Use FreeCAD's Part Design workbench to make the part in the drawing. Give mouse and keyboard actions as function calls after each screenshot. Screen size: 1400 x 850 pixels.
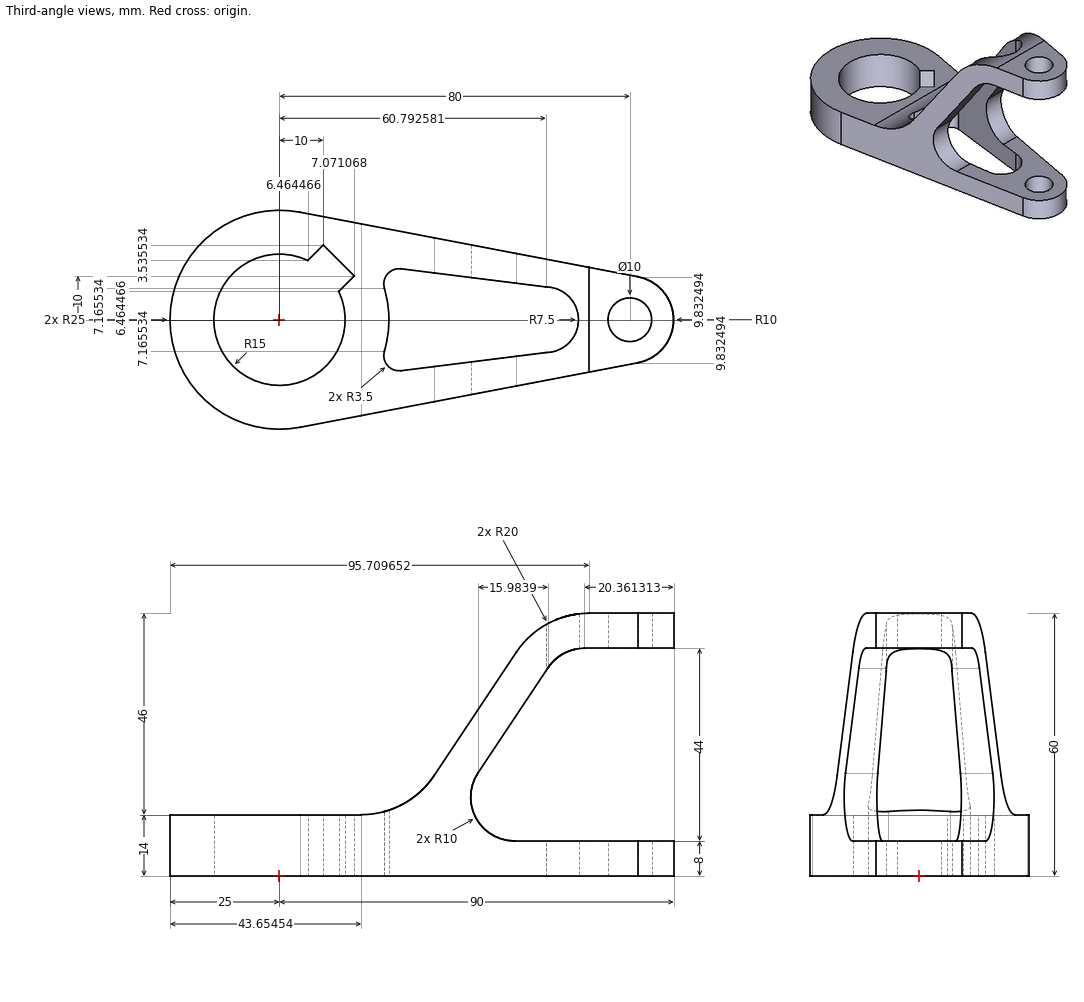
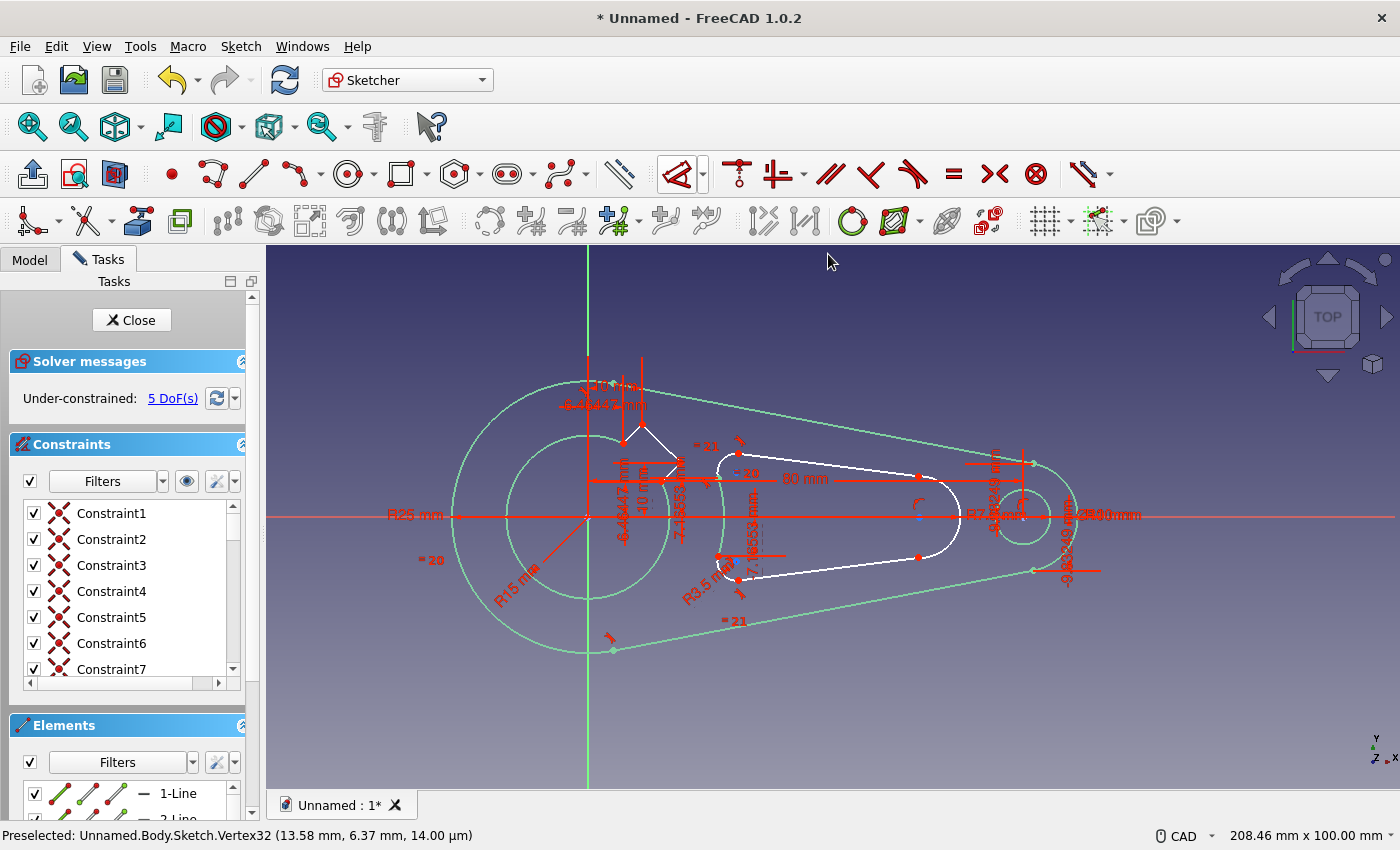
scroll(631, 436, up, 4)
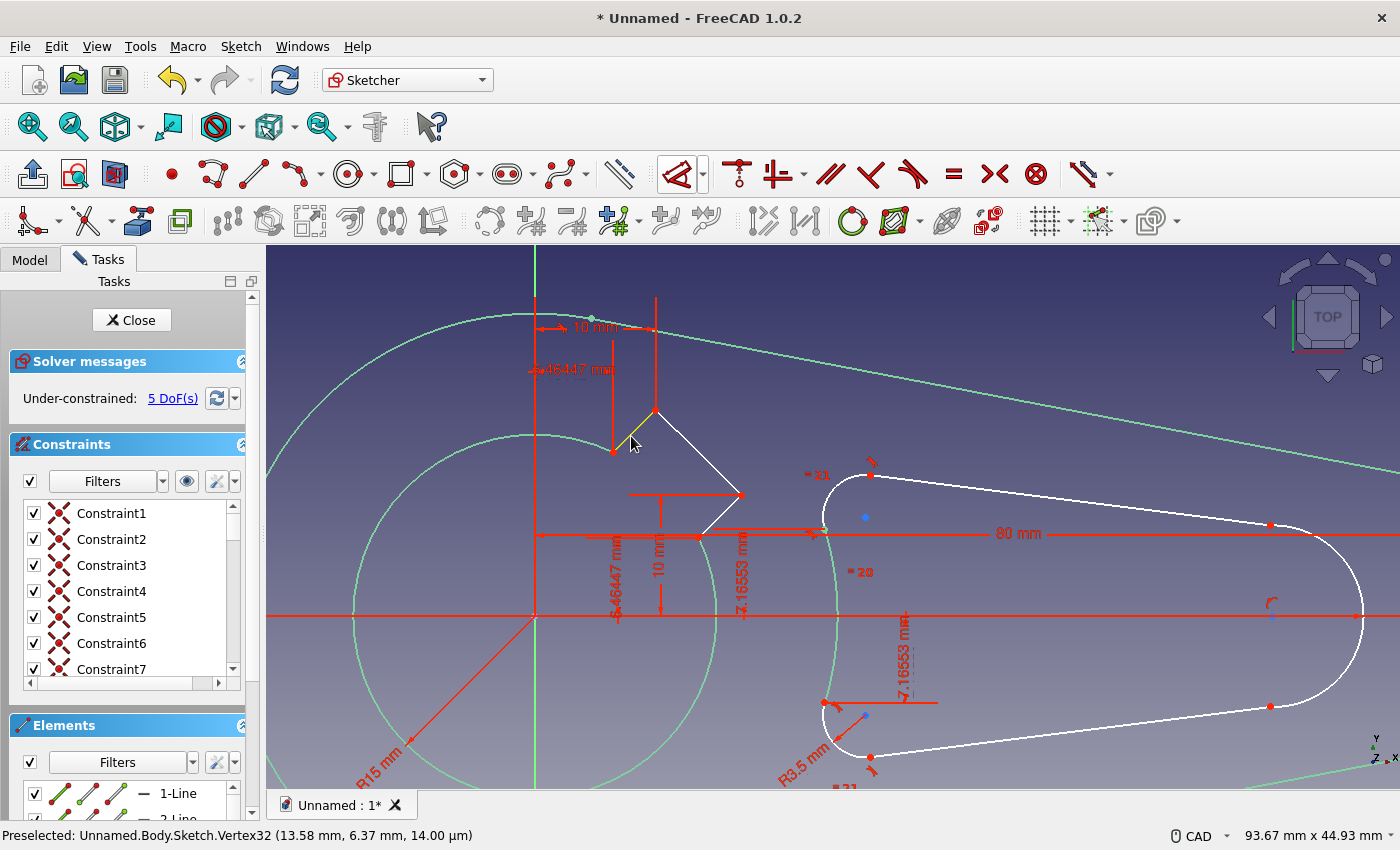
click(630, 435)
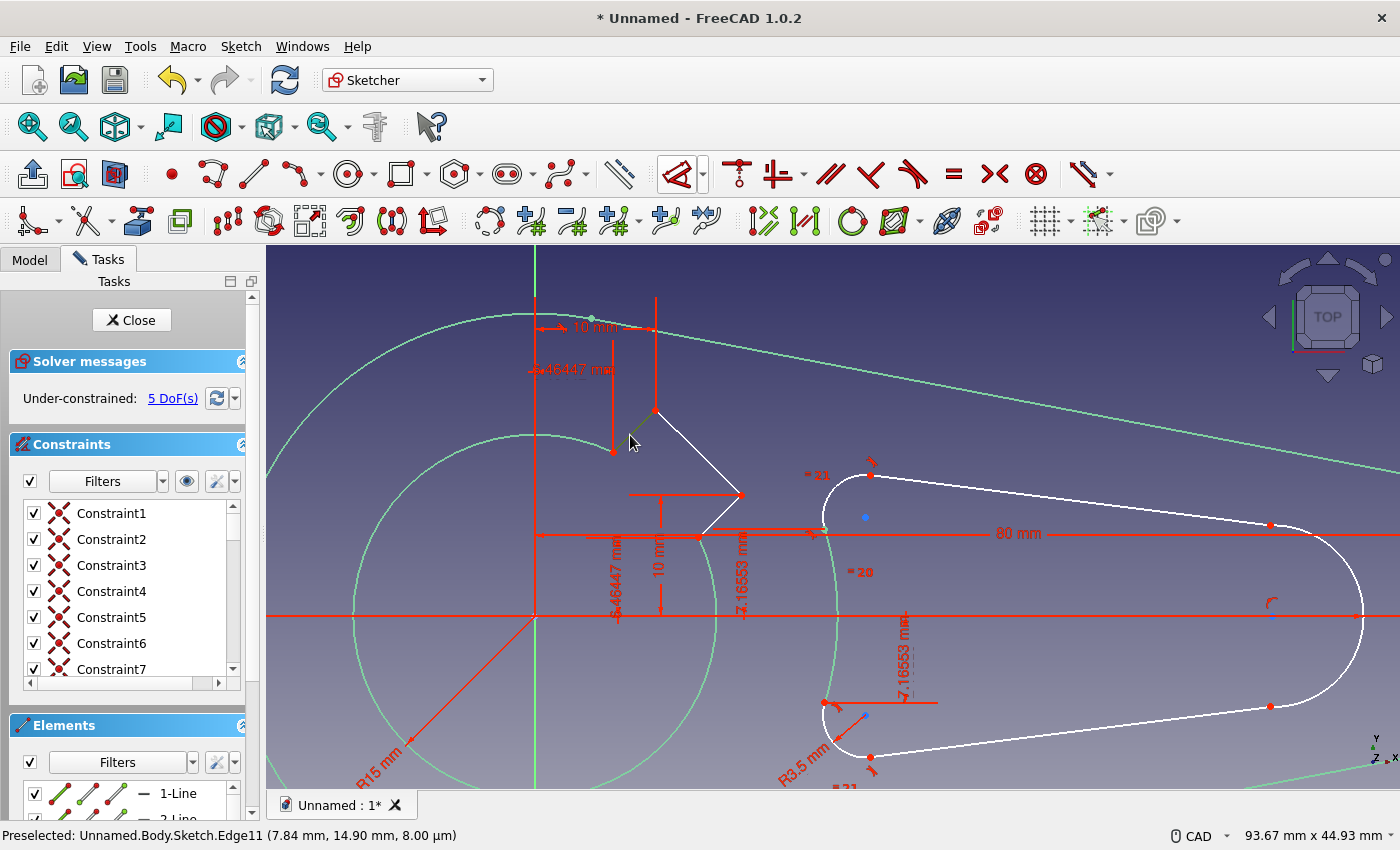
click(702, 174)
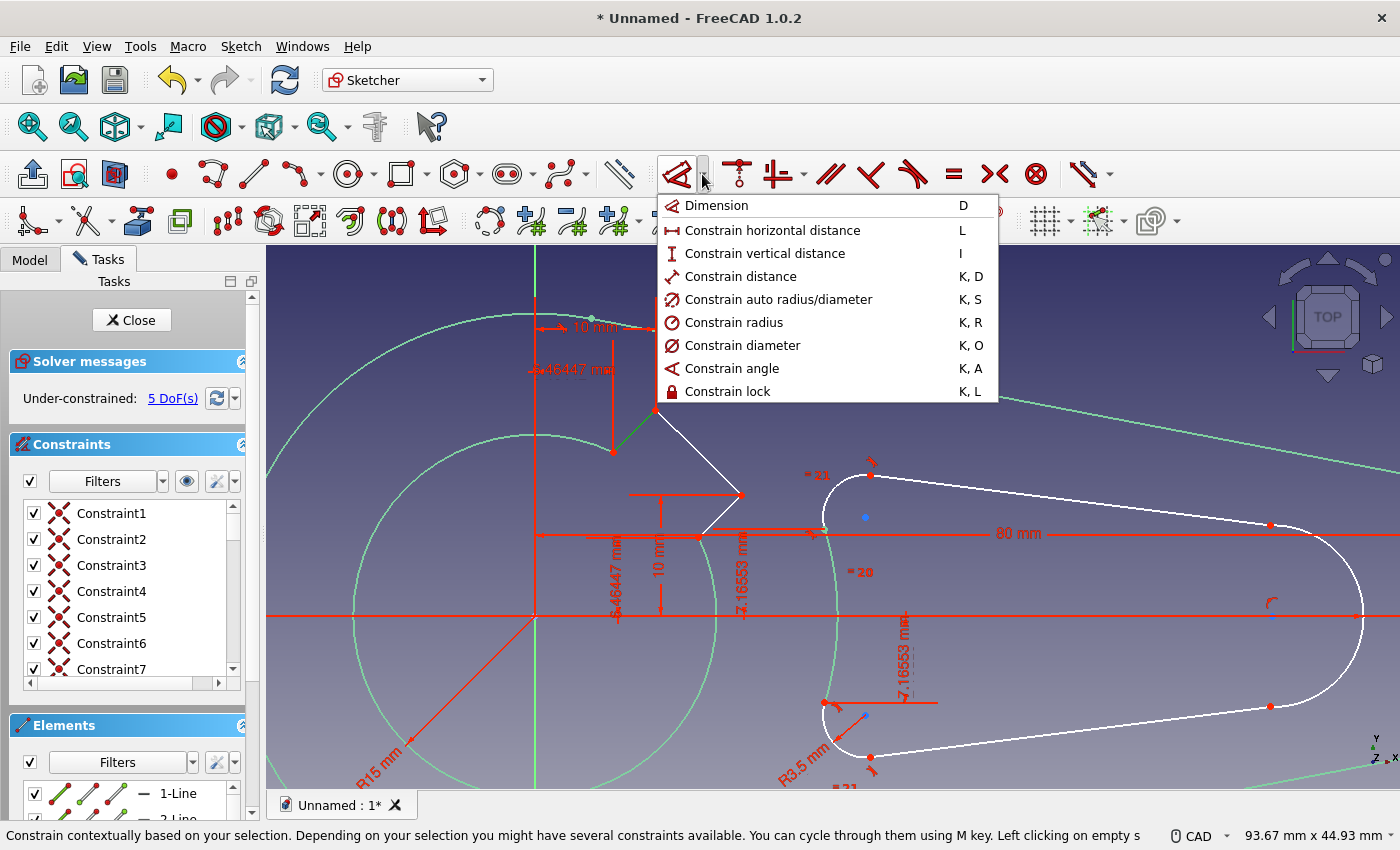
click(828, 254)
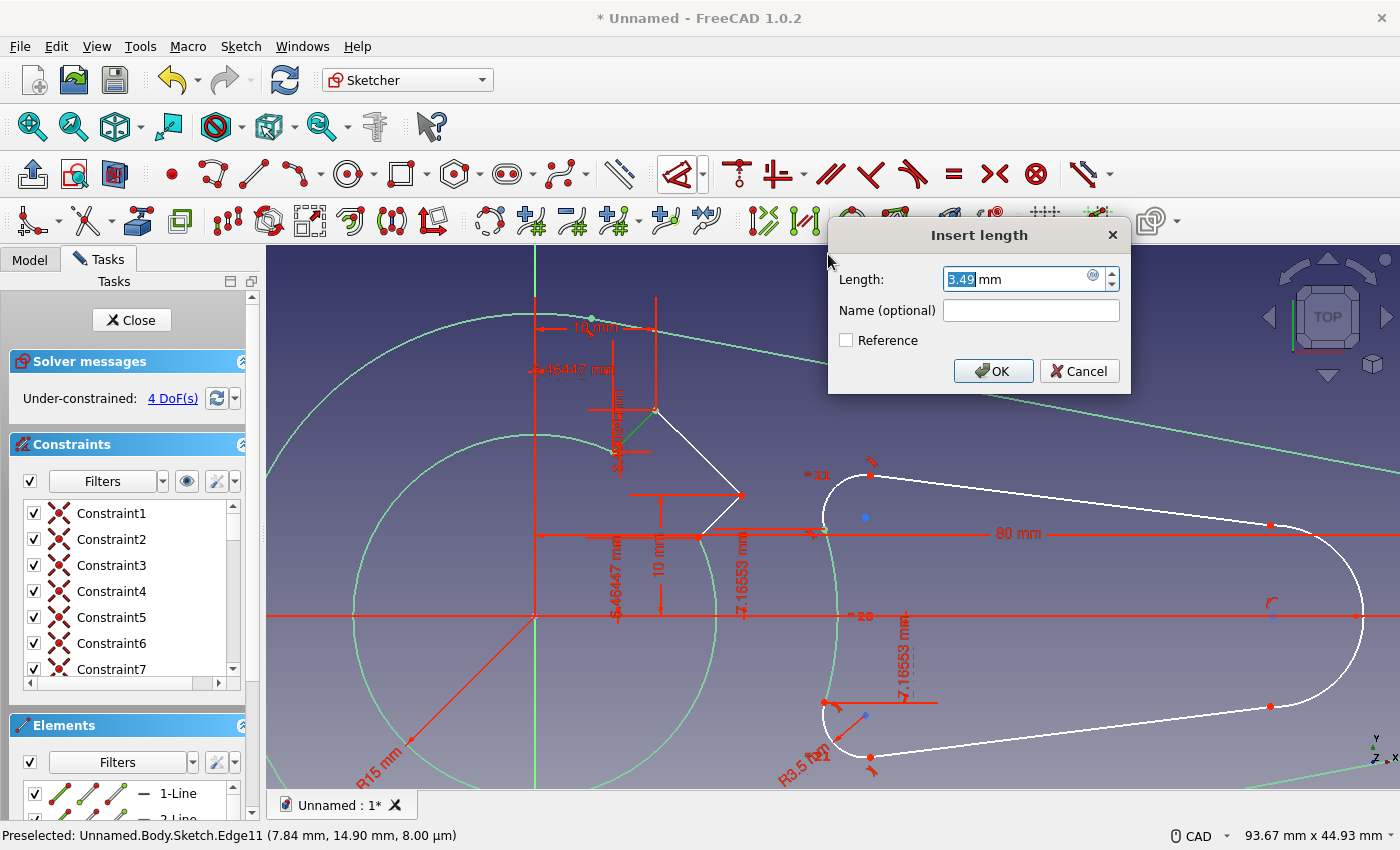
text(3.535534)
key(Return)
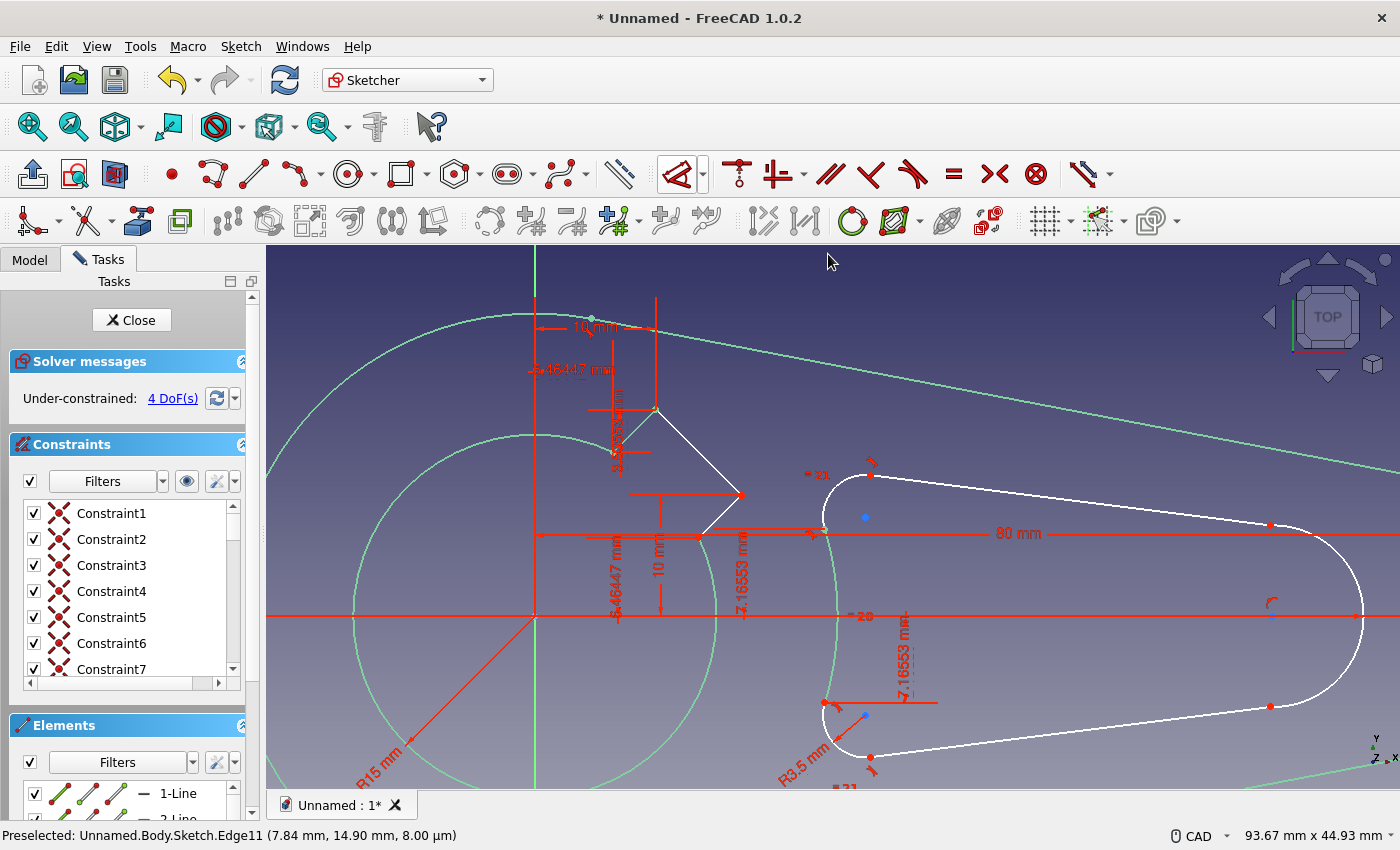
click(682, 435)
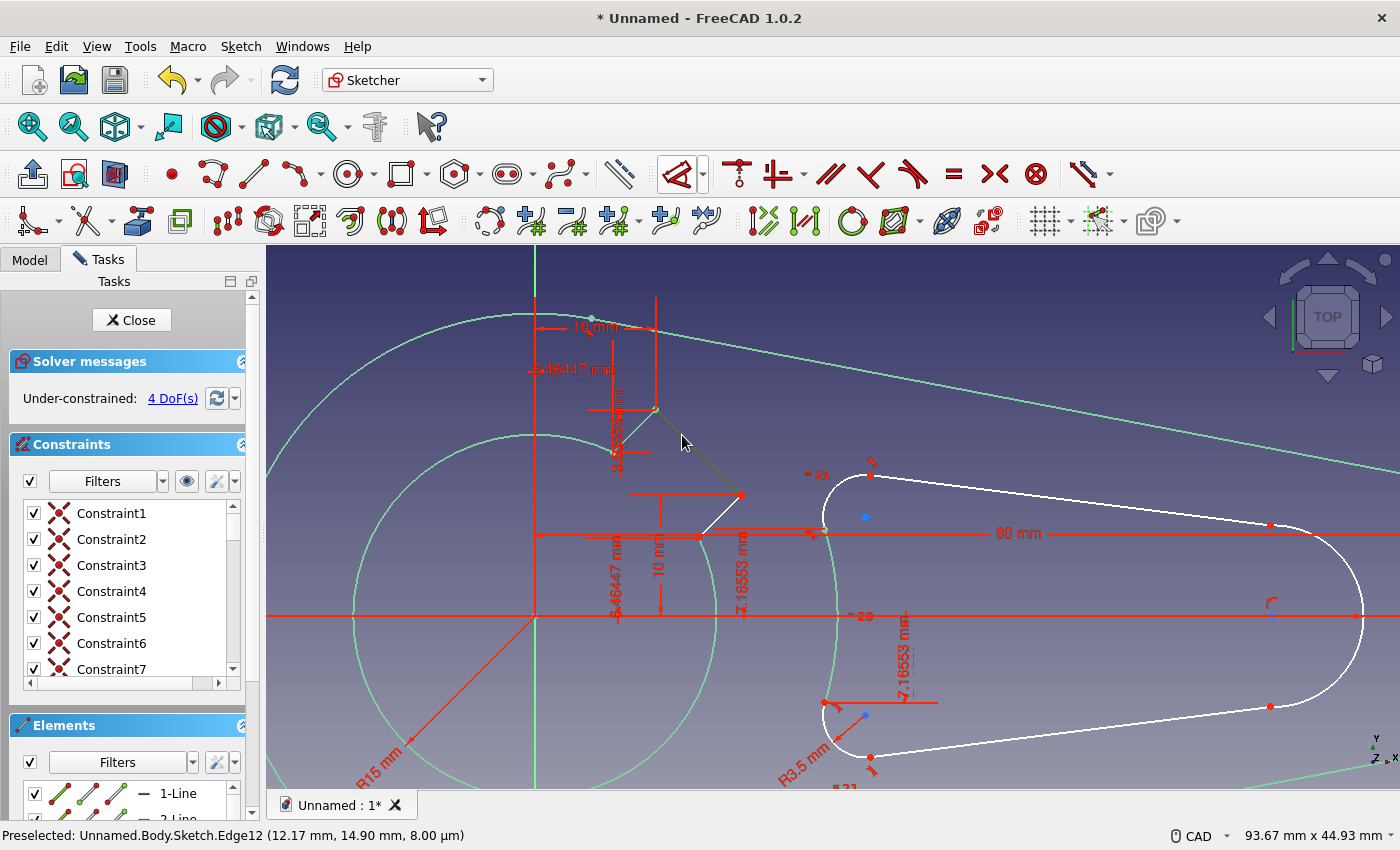
click(702, 174)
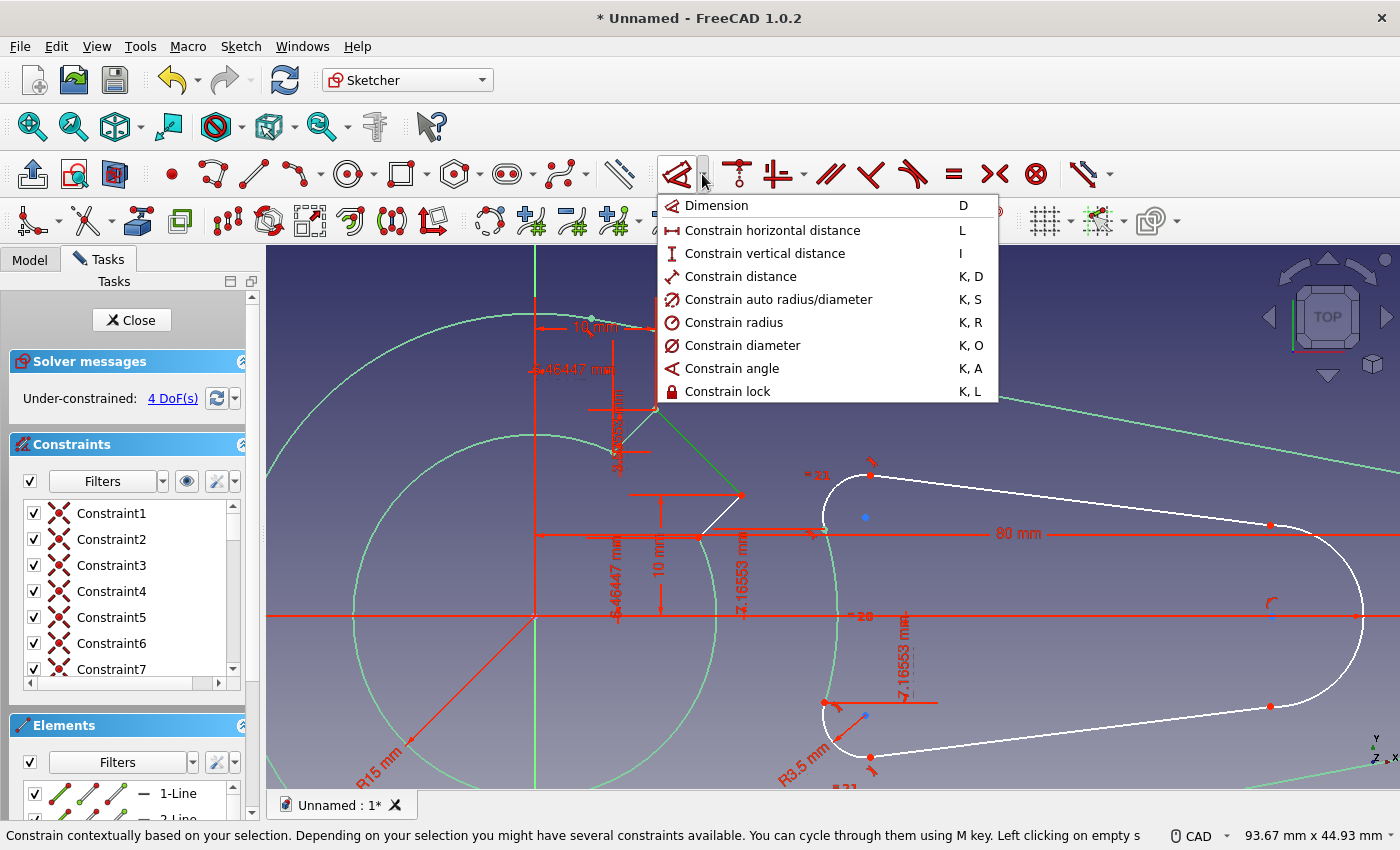
click(828, 230)